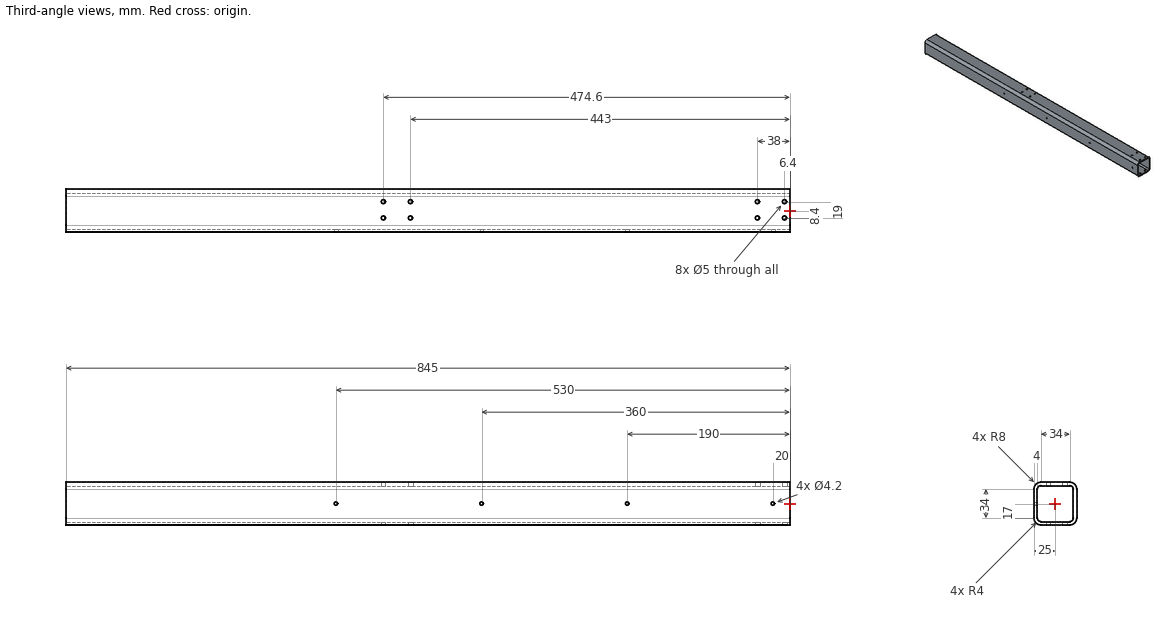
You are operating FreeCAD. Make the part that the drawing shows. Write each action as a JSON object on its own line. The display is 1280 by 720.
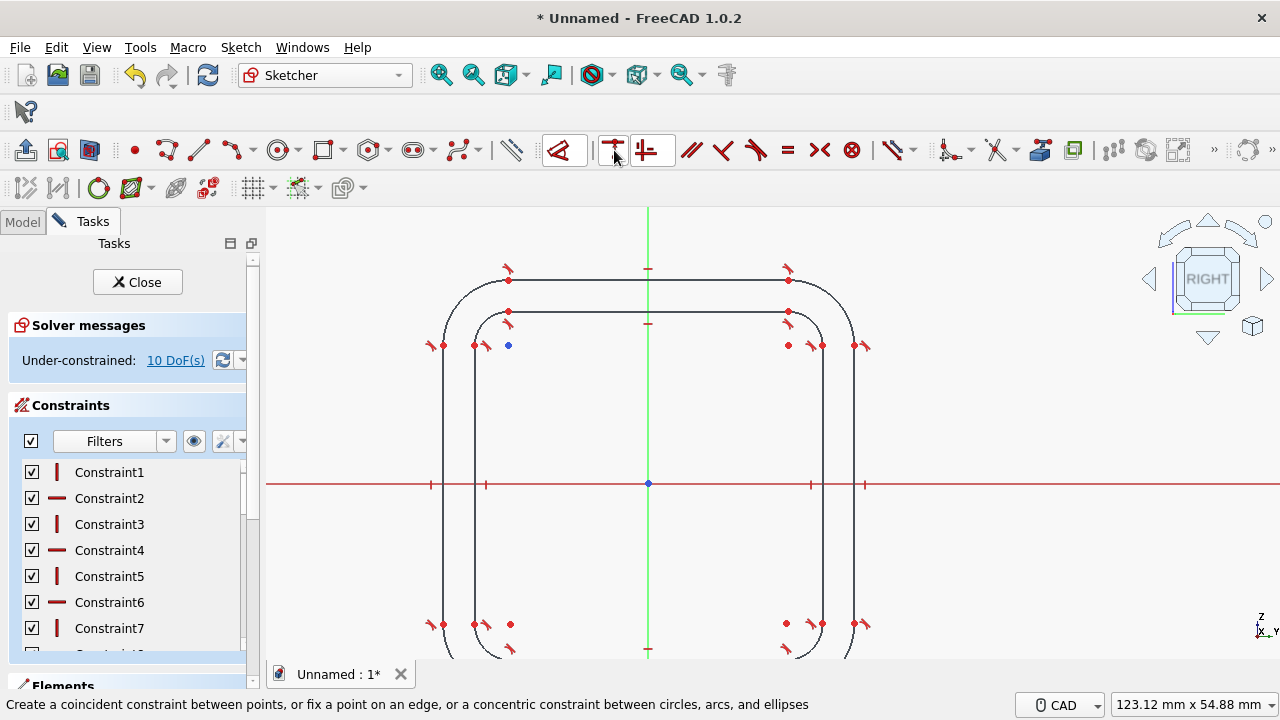
{"action": "left_click", "coordinate": [479, 287]}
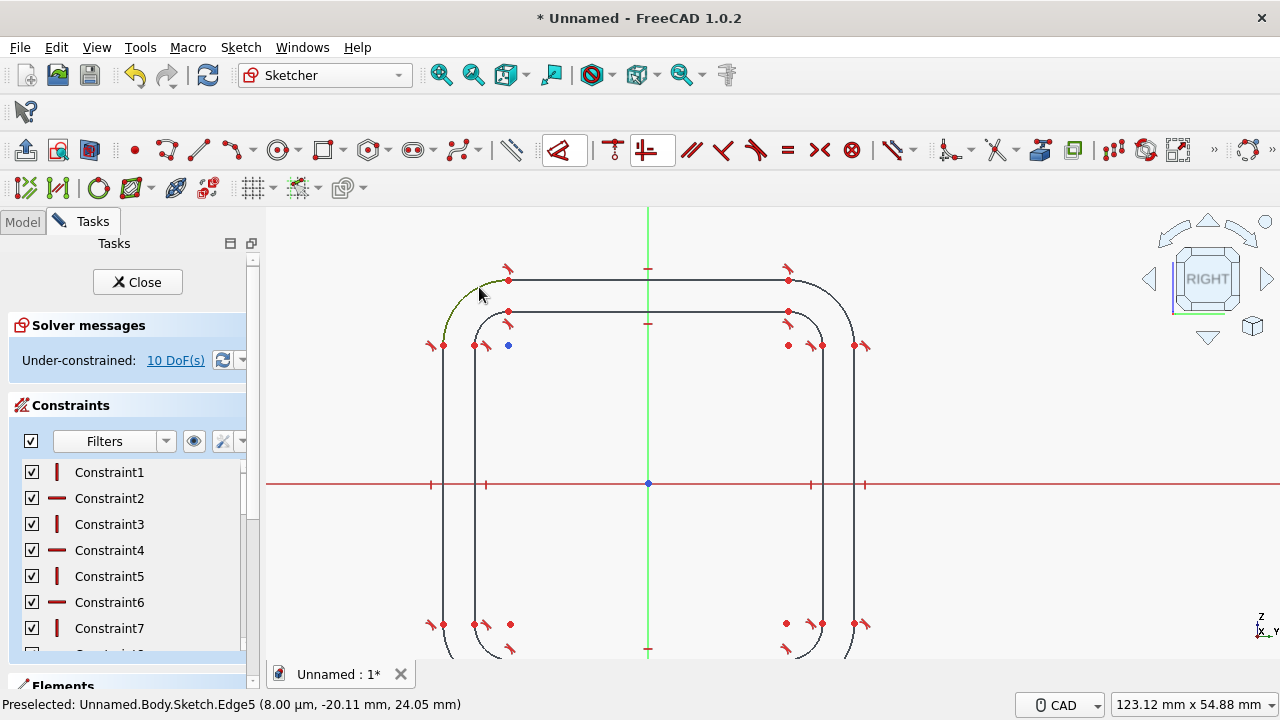
{"action": "left_click", "coordinate": [847, 316]}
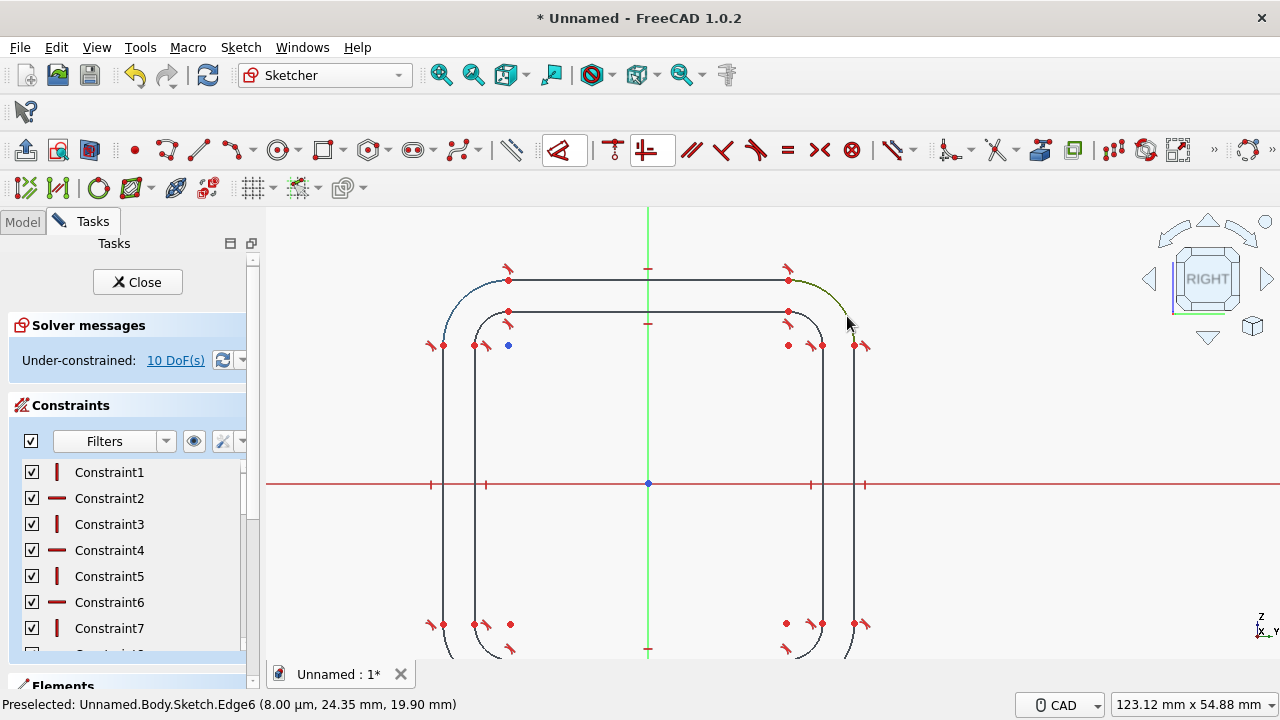
{"action": "scroll", "coordinate": [819, 330], "scroll_direction": "down", "scroll_amount": 2}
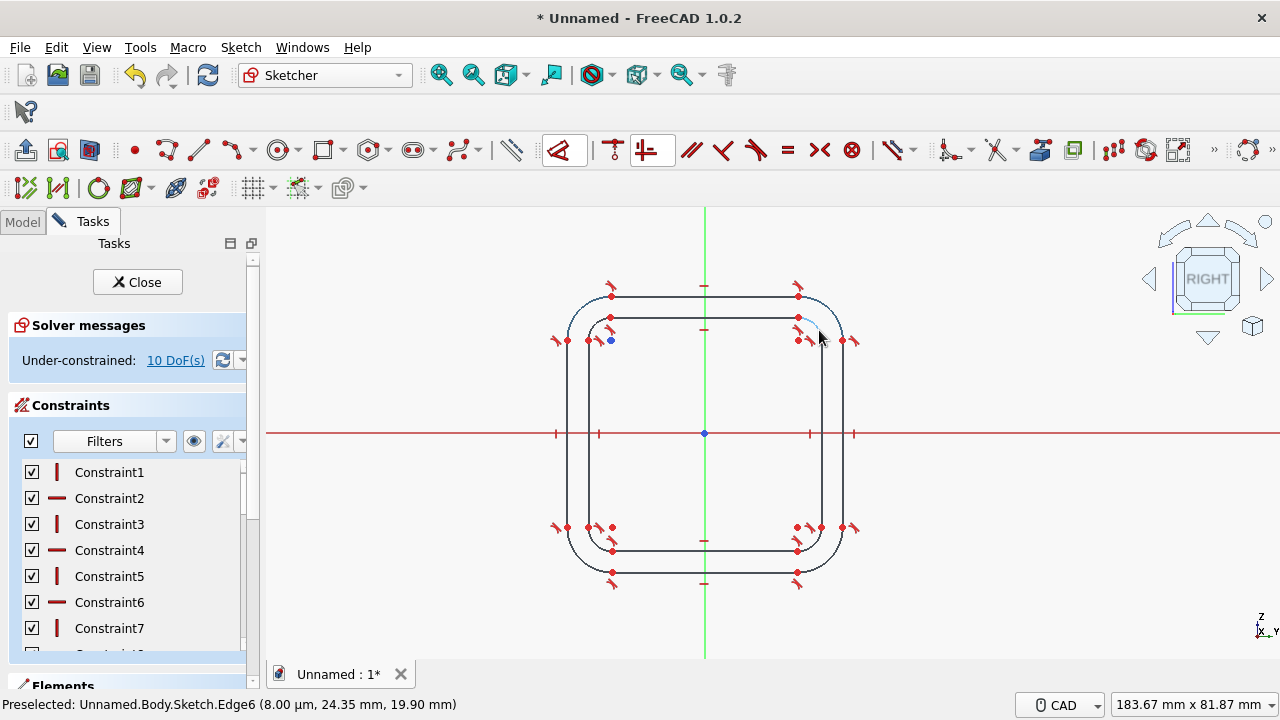
{"action": "left_click", "coordinate": [818, 568]}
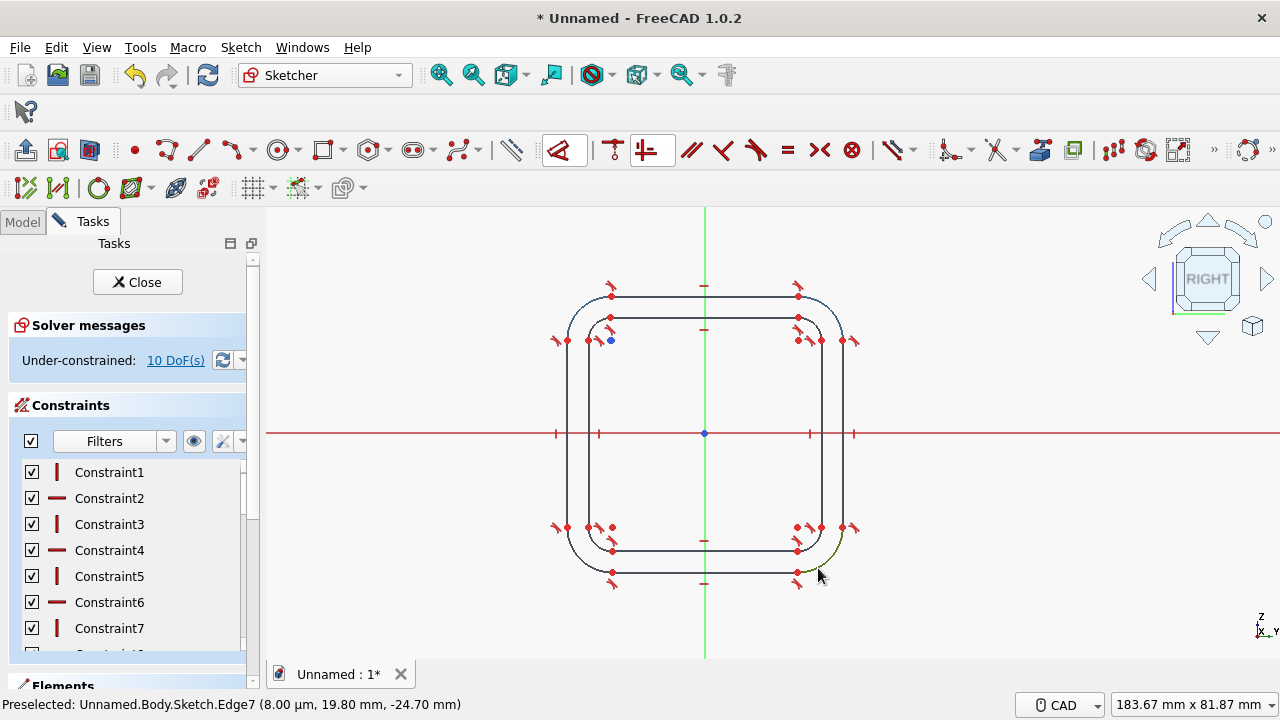
{"action": "left_click", "coordinate": [572, 548]}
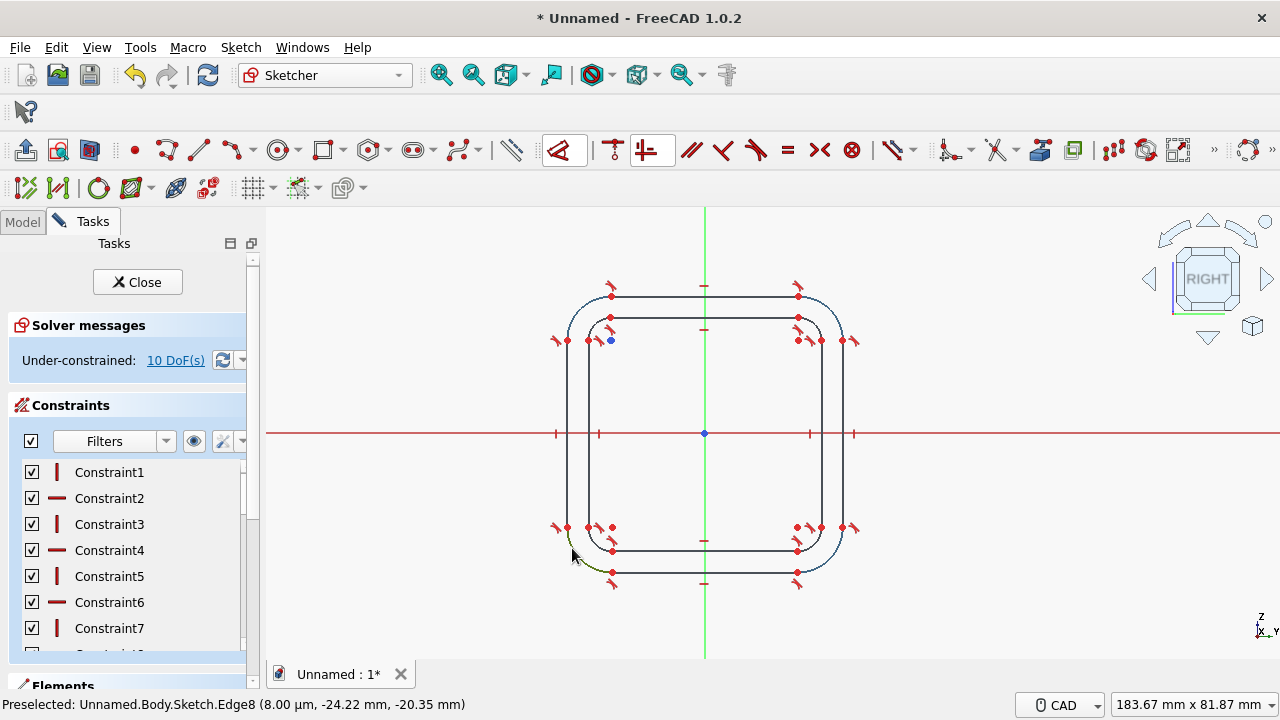
{"action": "left_click", "coordinate": [788, 150]}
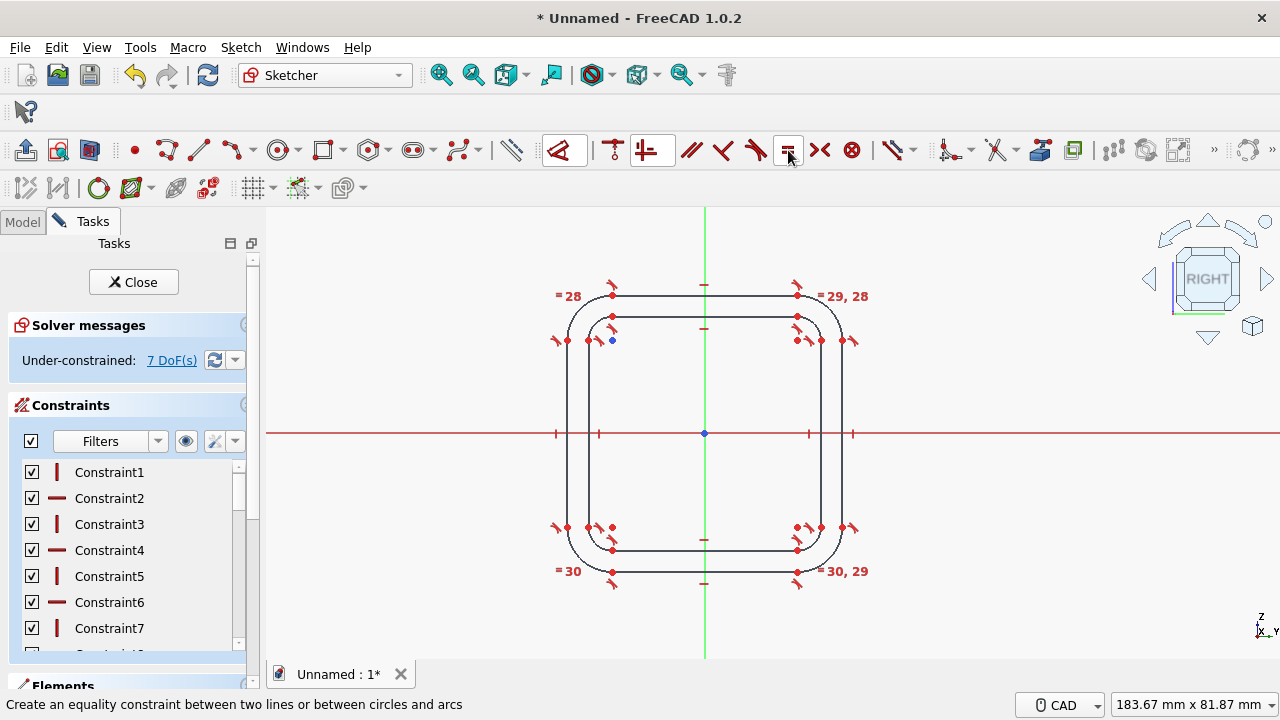
{"action": "scroll", "coordinate": [591, 538], "scroll_direction": "up", "scroll_amount": 2}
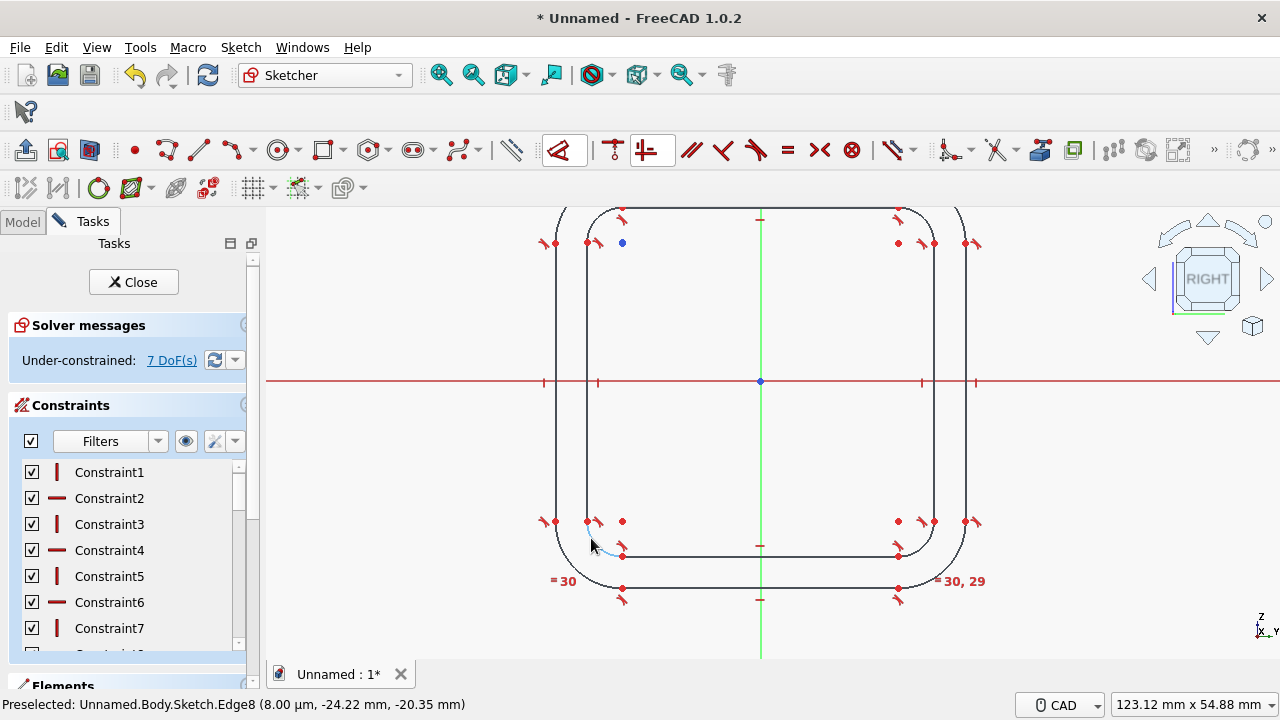
{"action": "left_click", "coordinate": [591, 537]}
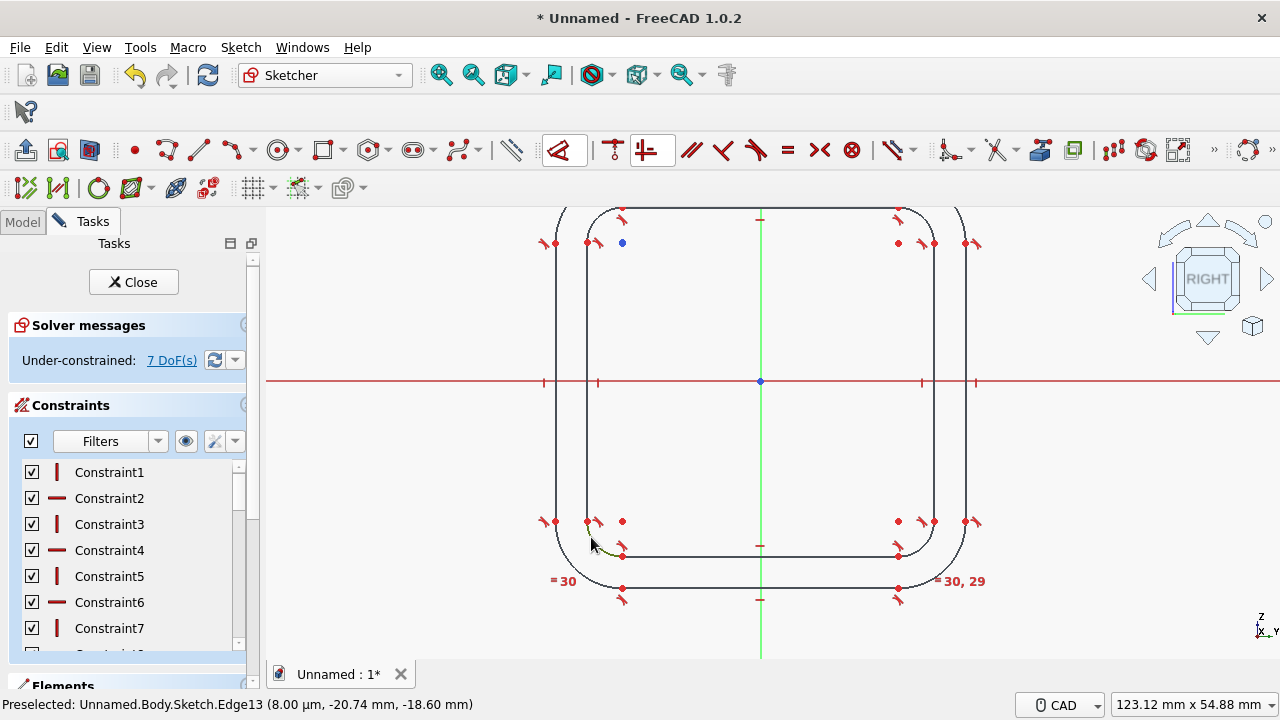
{"action": "scroll", "coordinate": [591, 539], "scroll_direction": "down", "scroll_amount": 2}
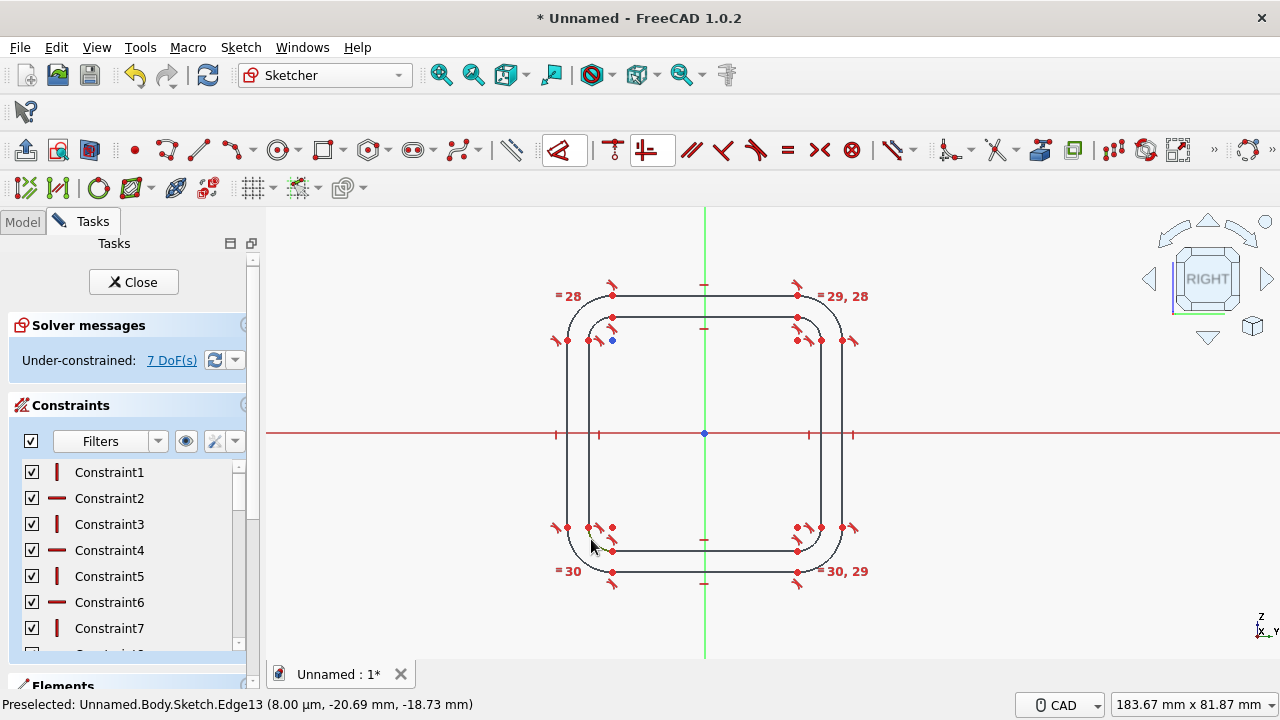
{"action": "scroll", "coordinate": [601, 320], "scroll_direction": "up", "scroll_amount": 2}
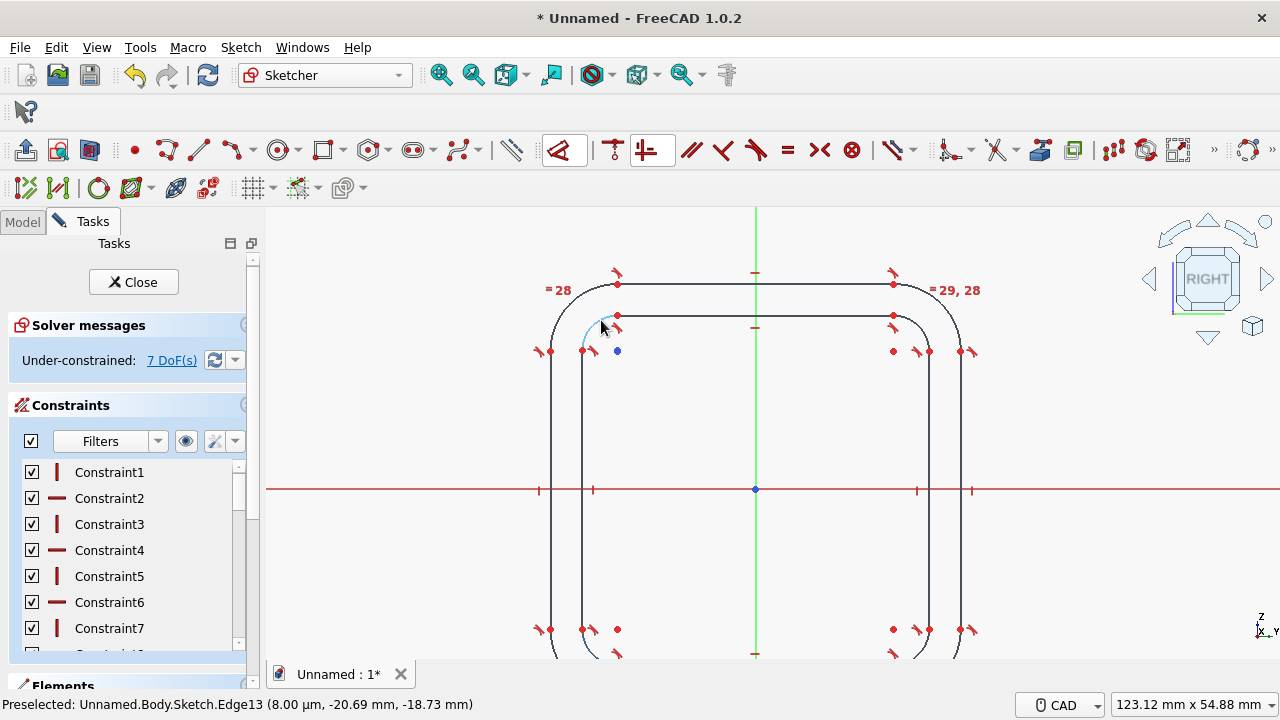
{"action": "left_click", "coordinate": [601, 320]}